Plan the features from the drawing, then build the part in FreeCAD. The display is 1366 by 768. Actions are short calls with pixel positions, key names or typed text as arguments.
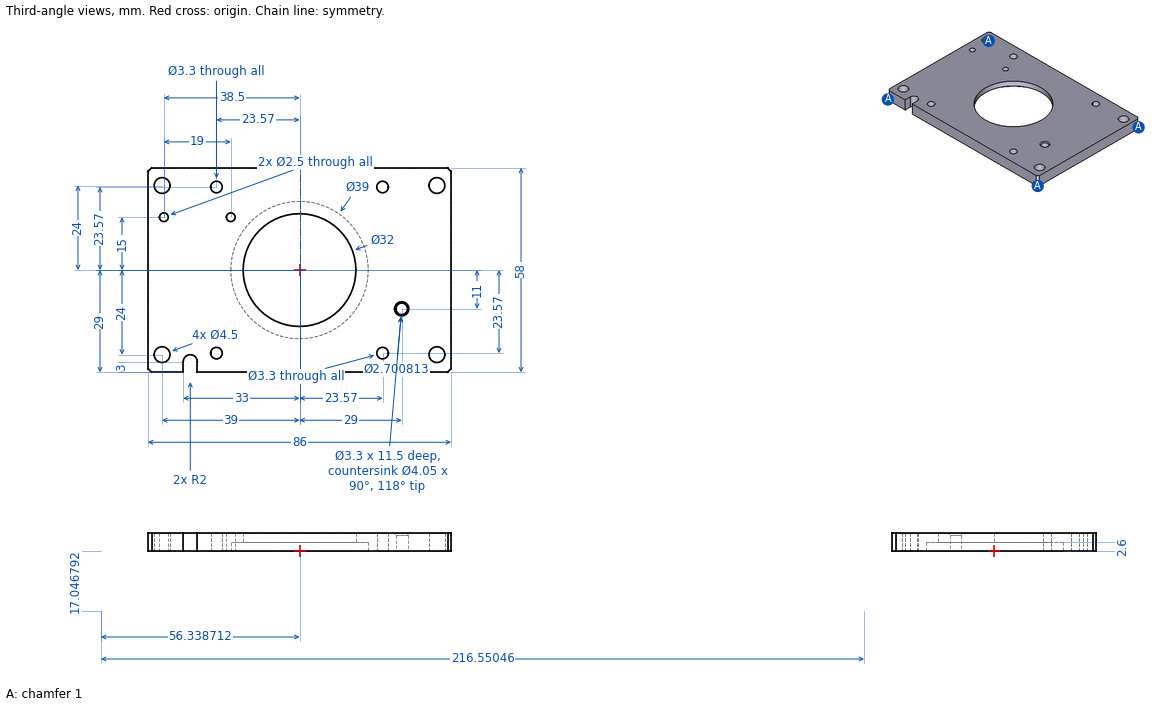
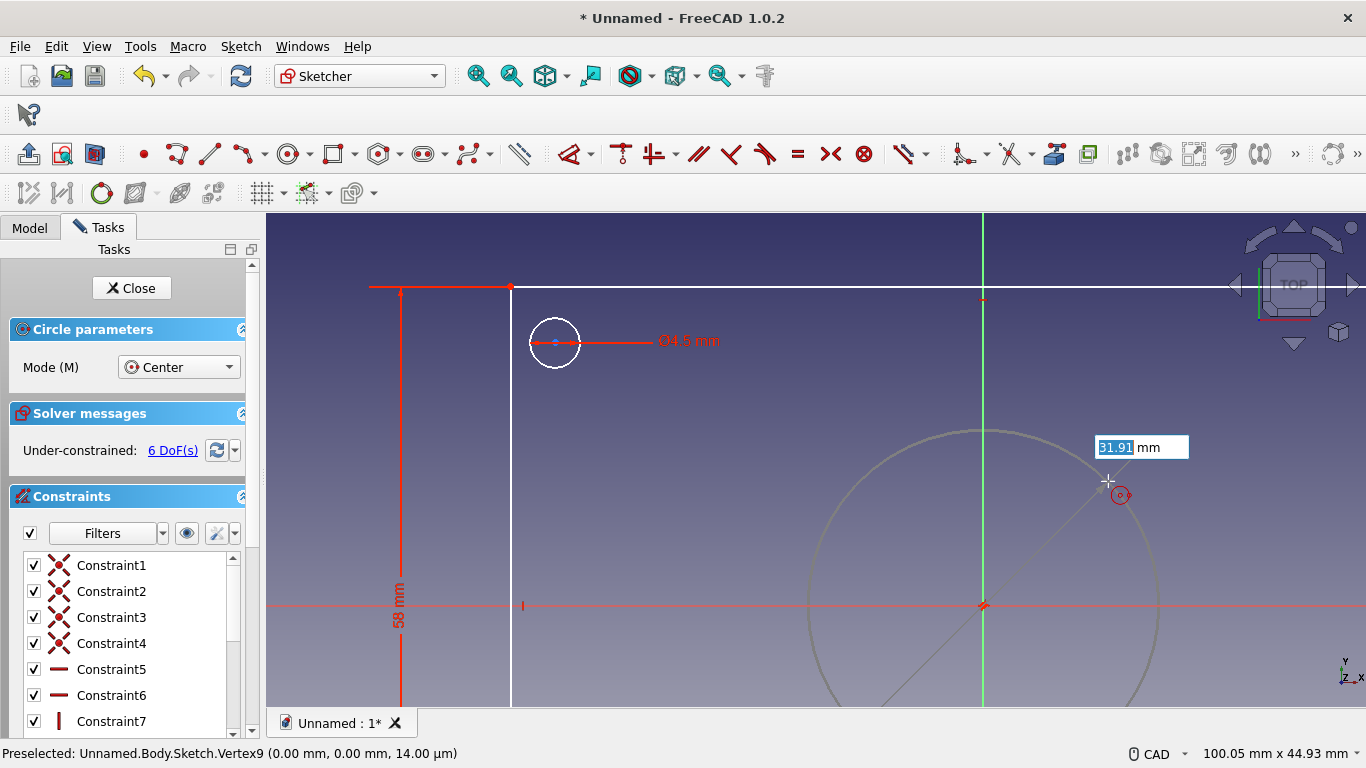
text(32)
key(Return)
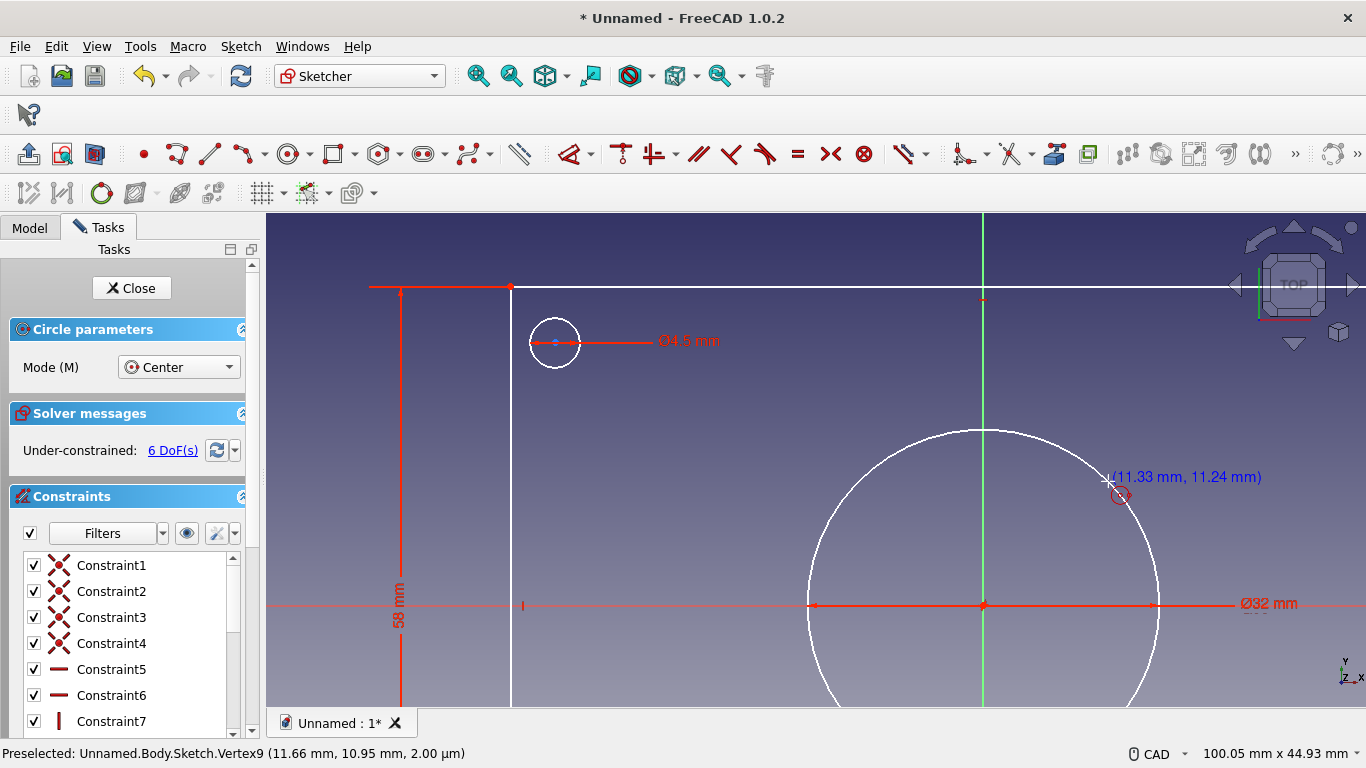
scroll(555, 341, down, 4)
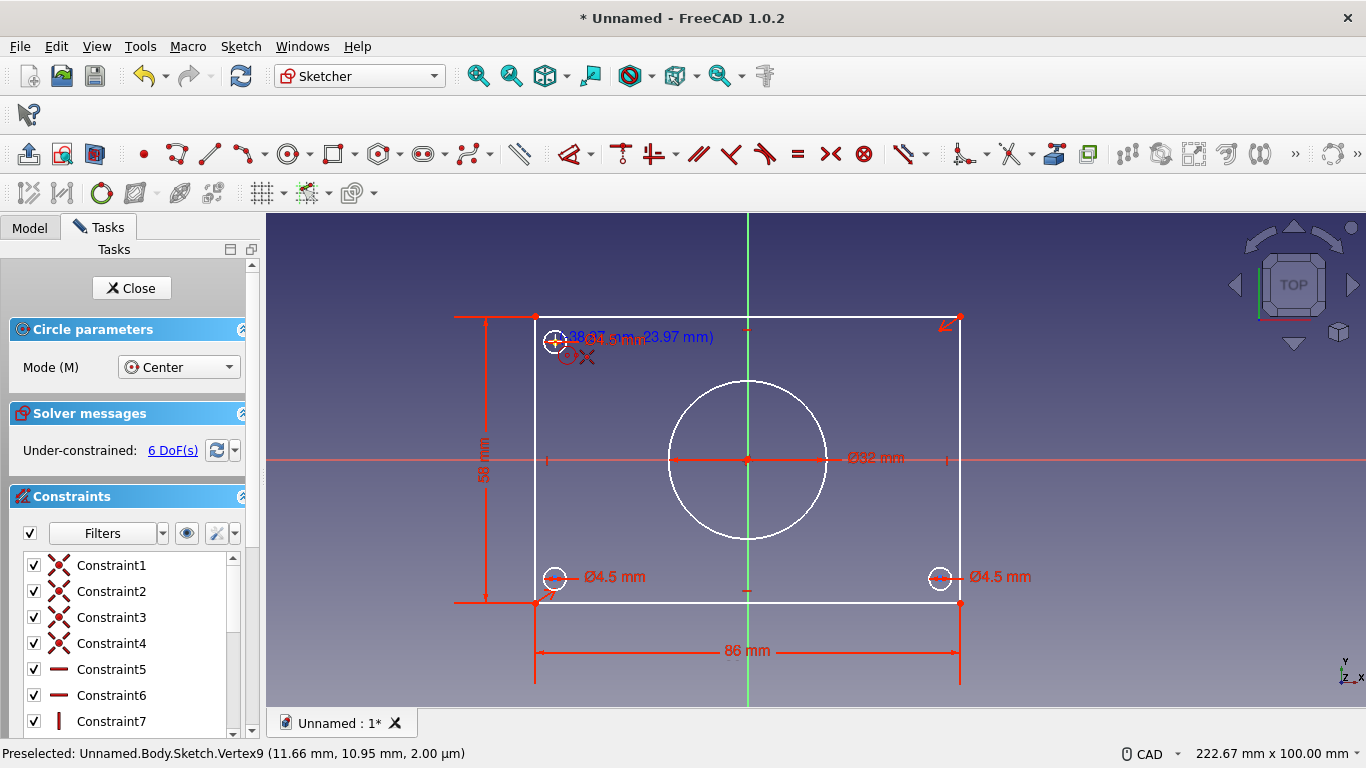
scroll(940, 341, up, 4)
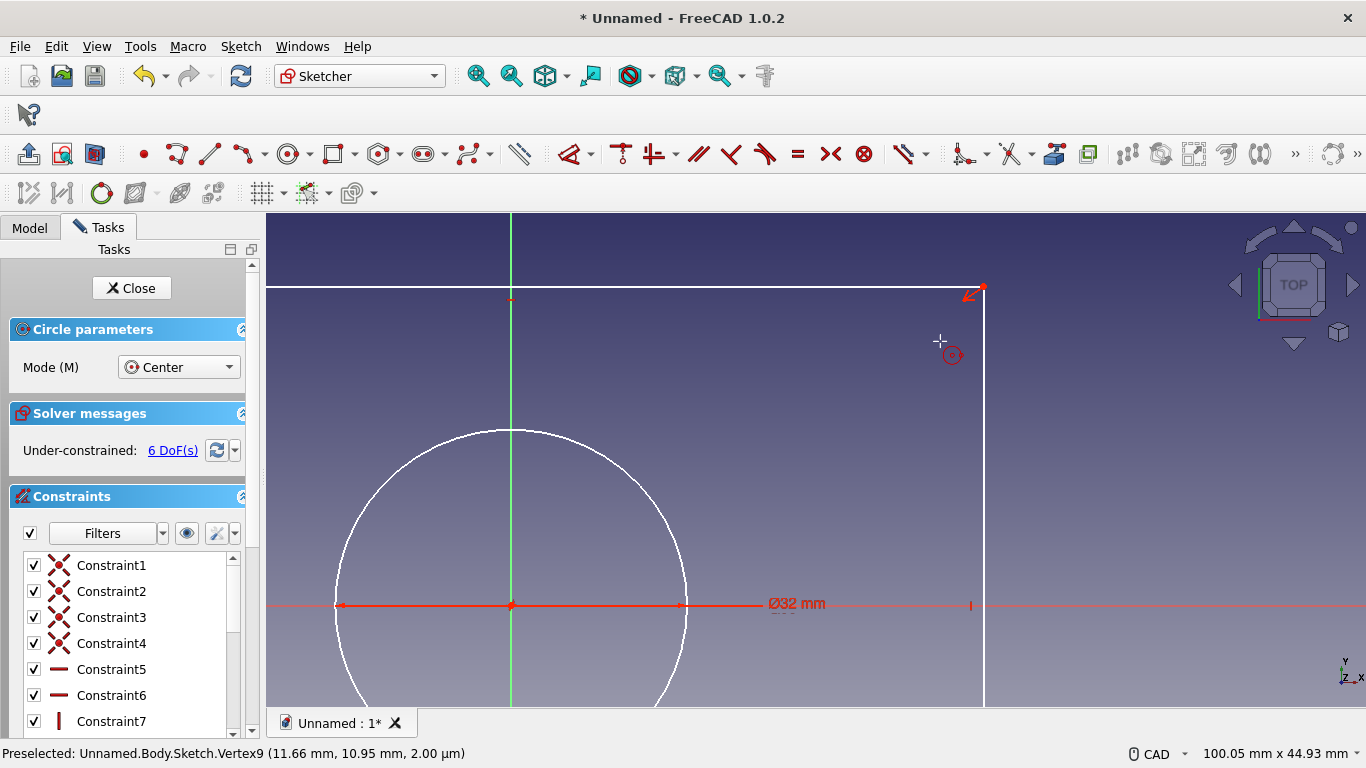
click(940, 342)
move(957, 324)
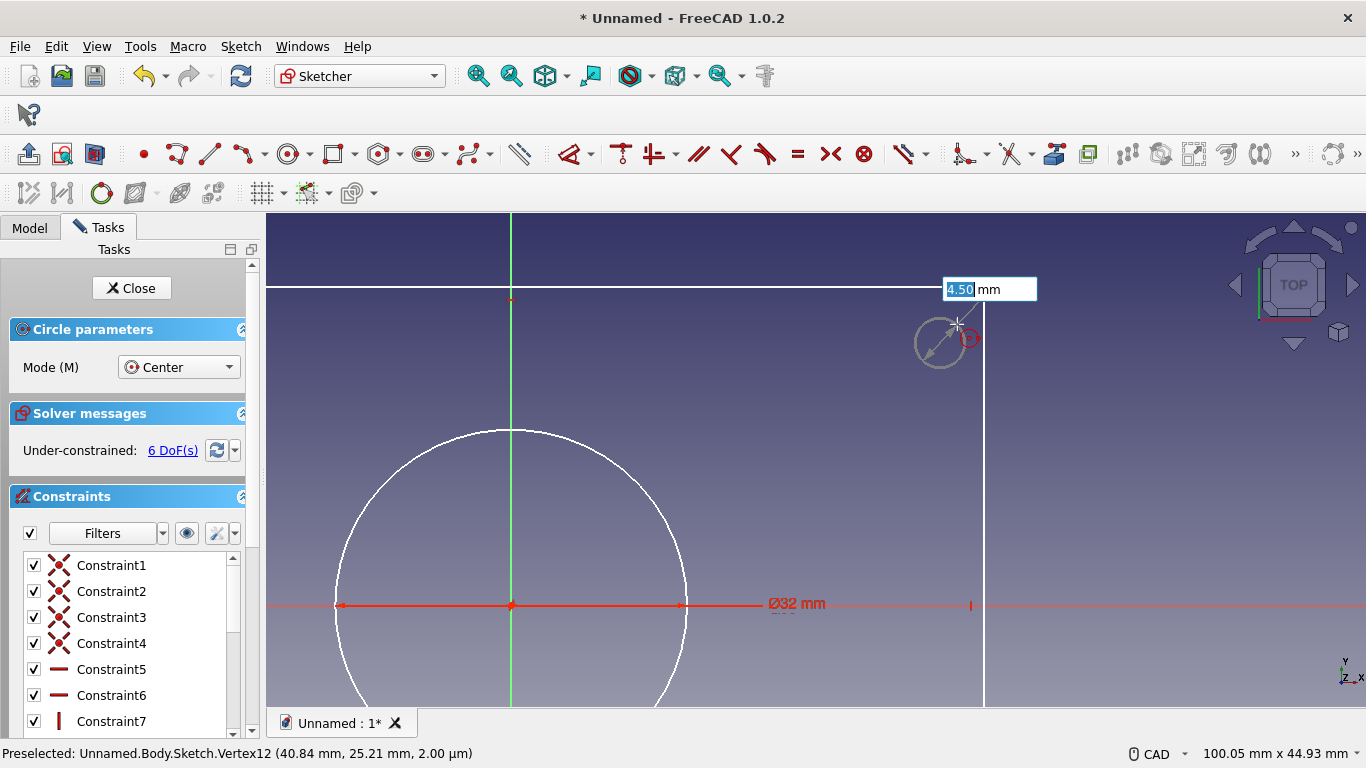
text(4.5)
key(Return)
key(Escape)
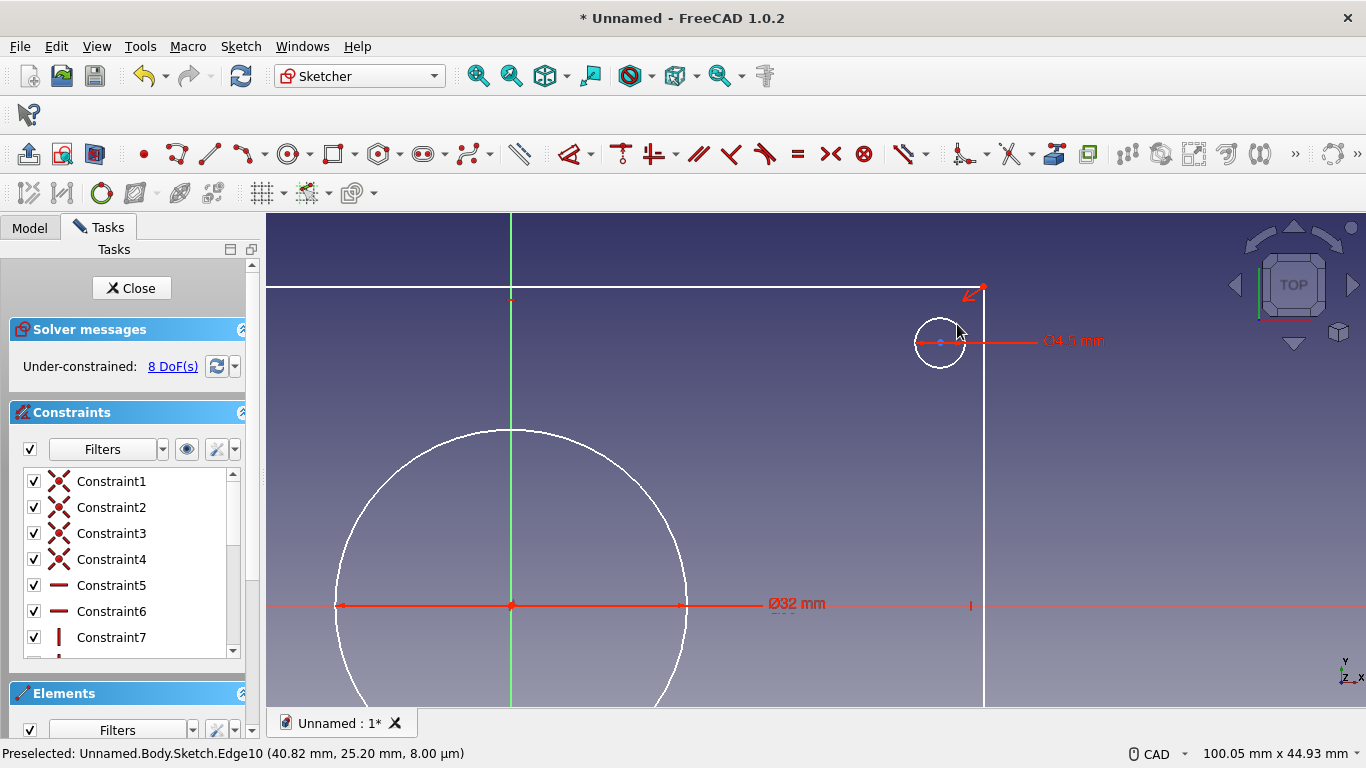
scroll(940, 341, down, 4)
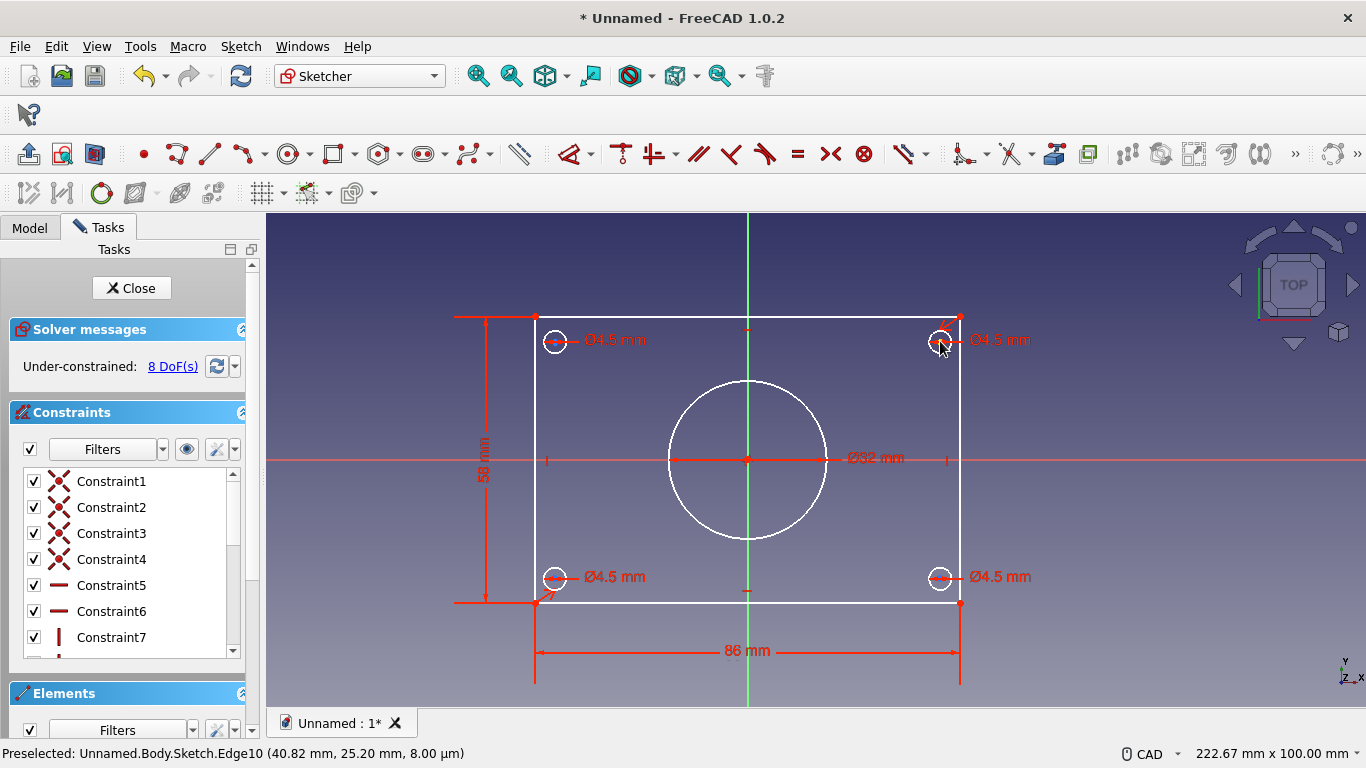
click(555, 579)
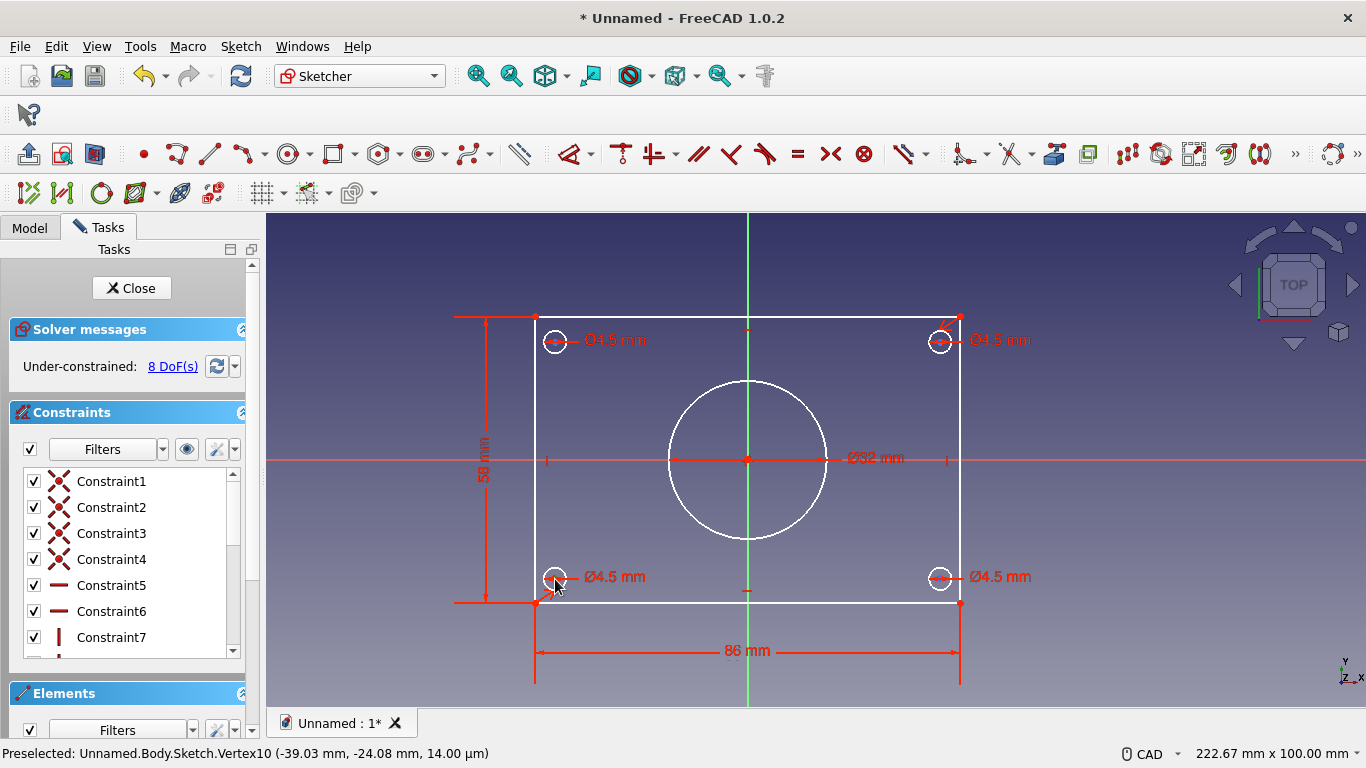
click(940, 579)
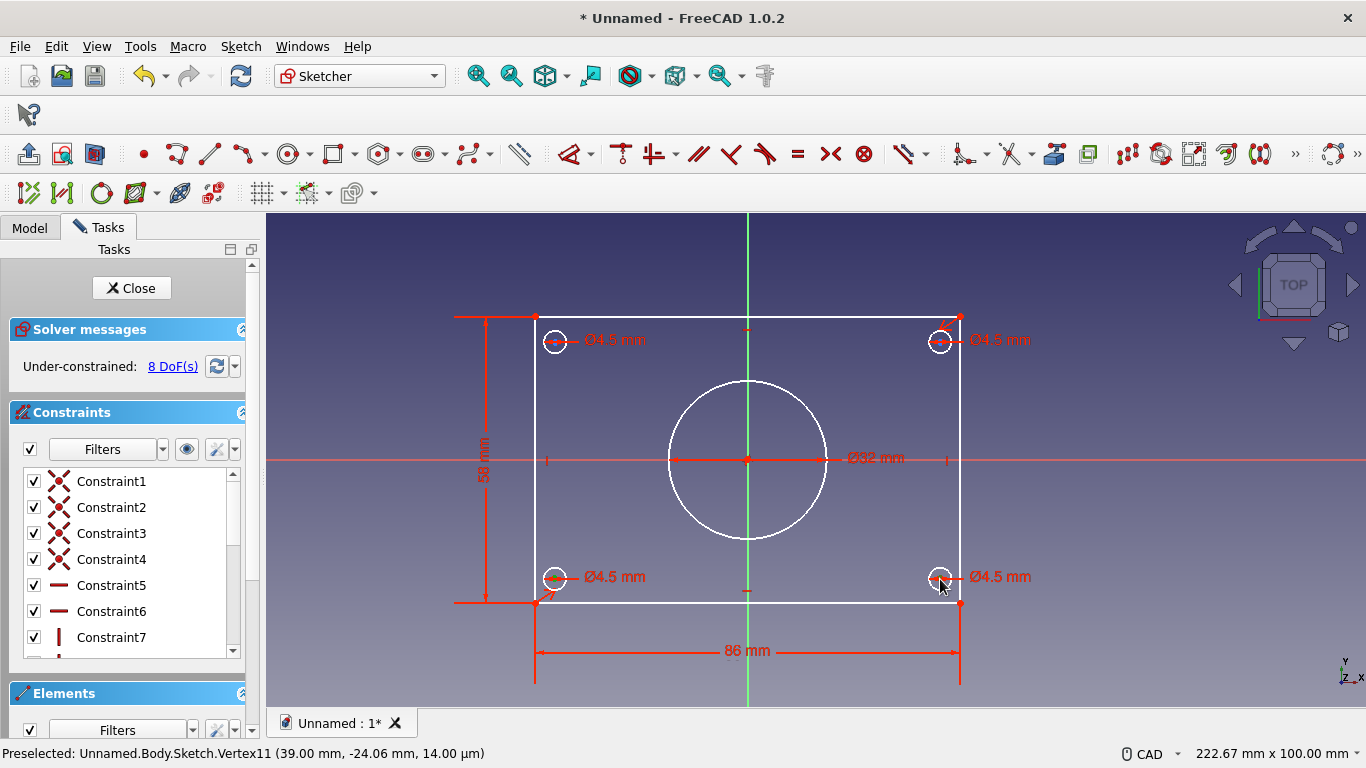
key(h)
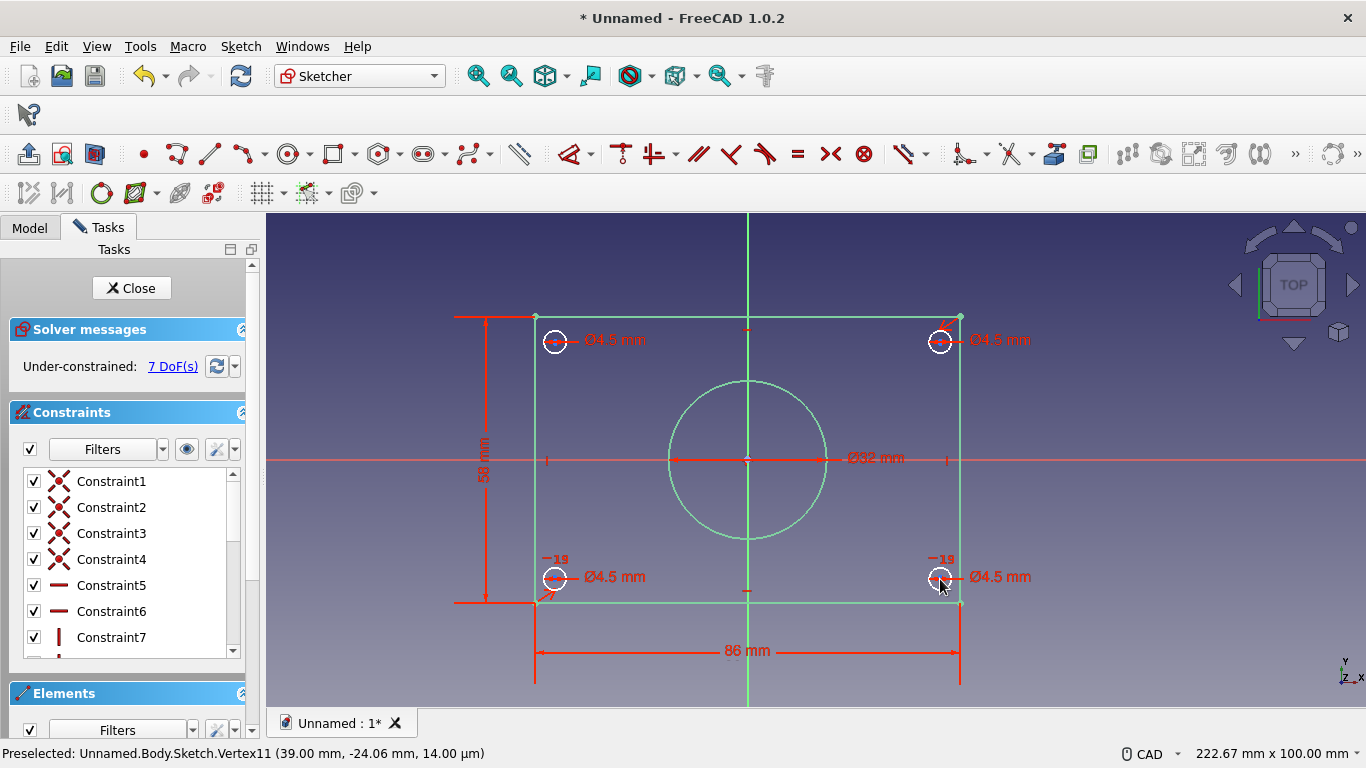
click(555, 579)